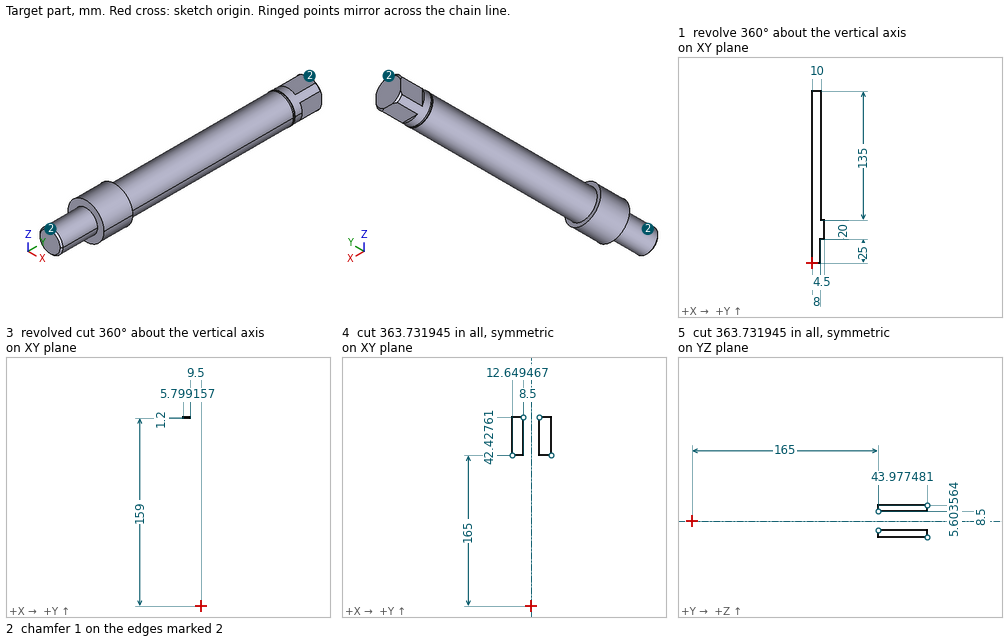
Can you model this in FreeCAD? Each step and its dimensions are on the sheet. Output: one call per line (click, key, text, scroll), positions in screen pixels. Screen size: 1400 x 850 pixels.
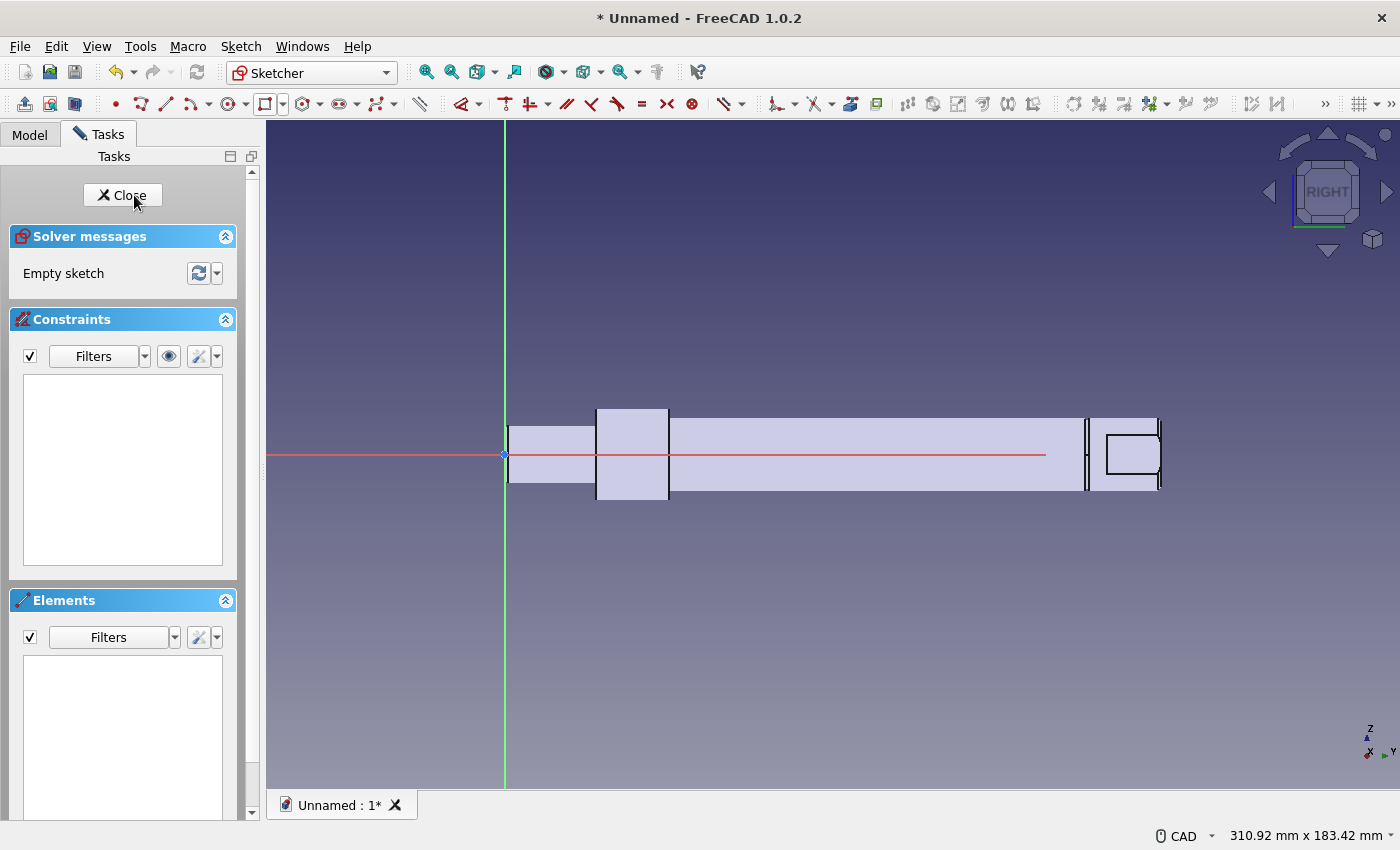
scroll(764, 454, down, 5)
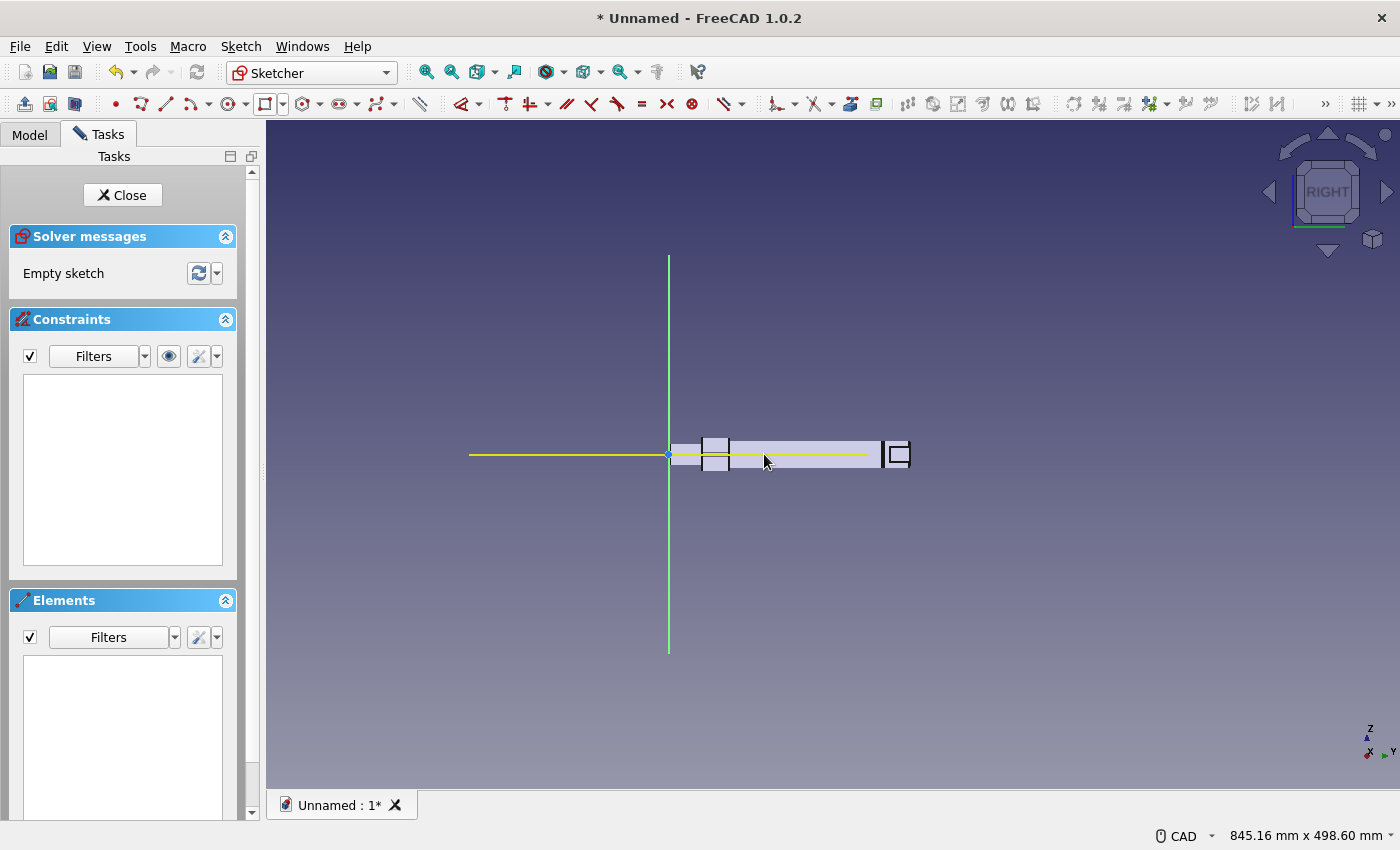
scroll(935, 454, up, 12)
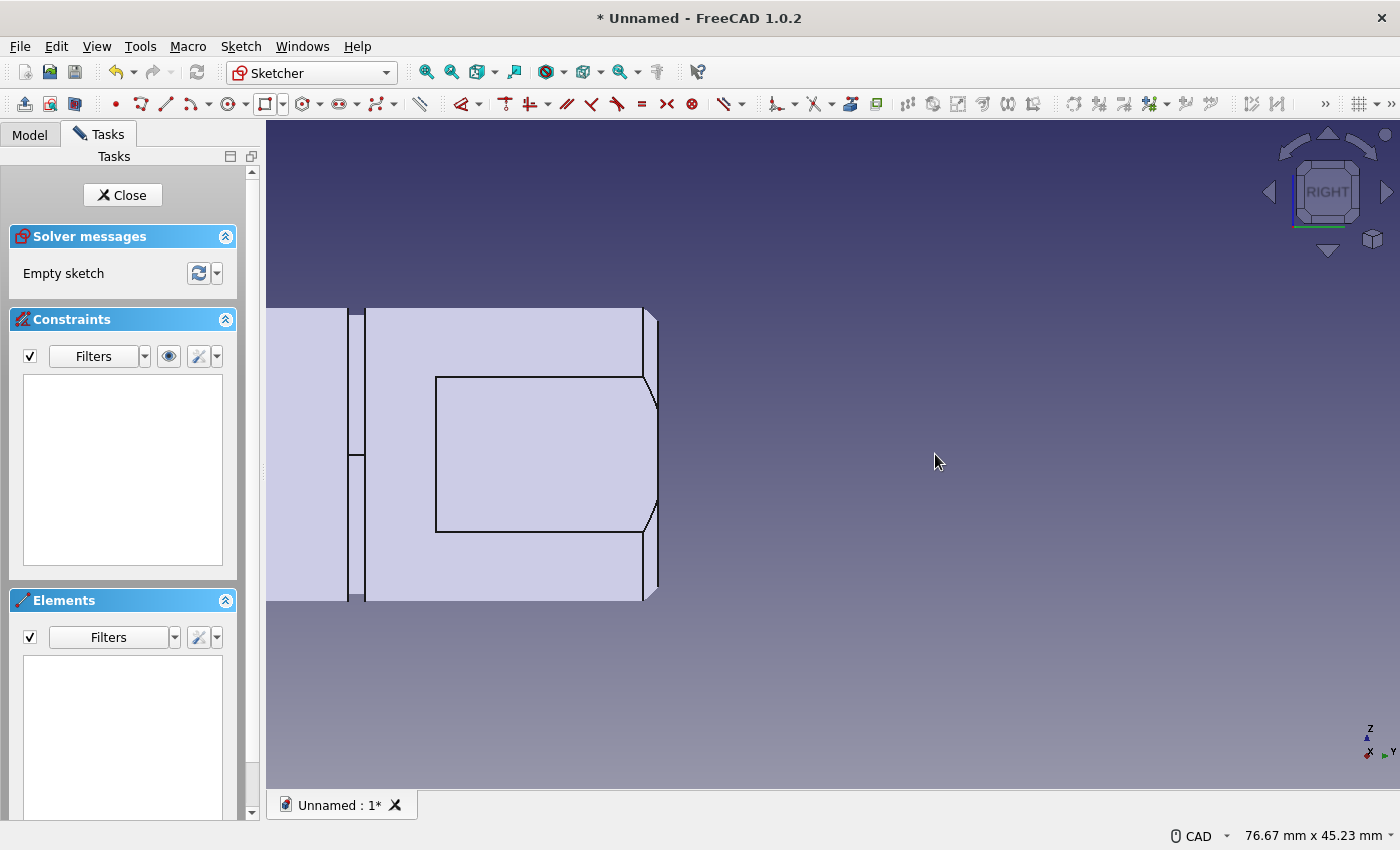
click(264, 104)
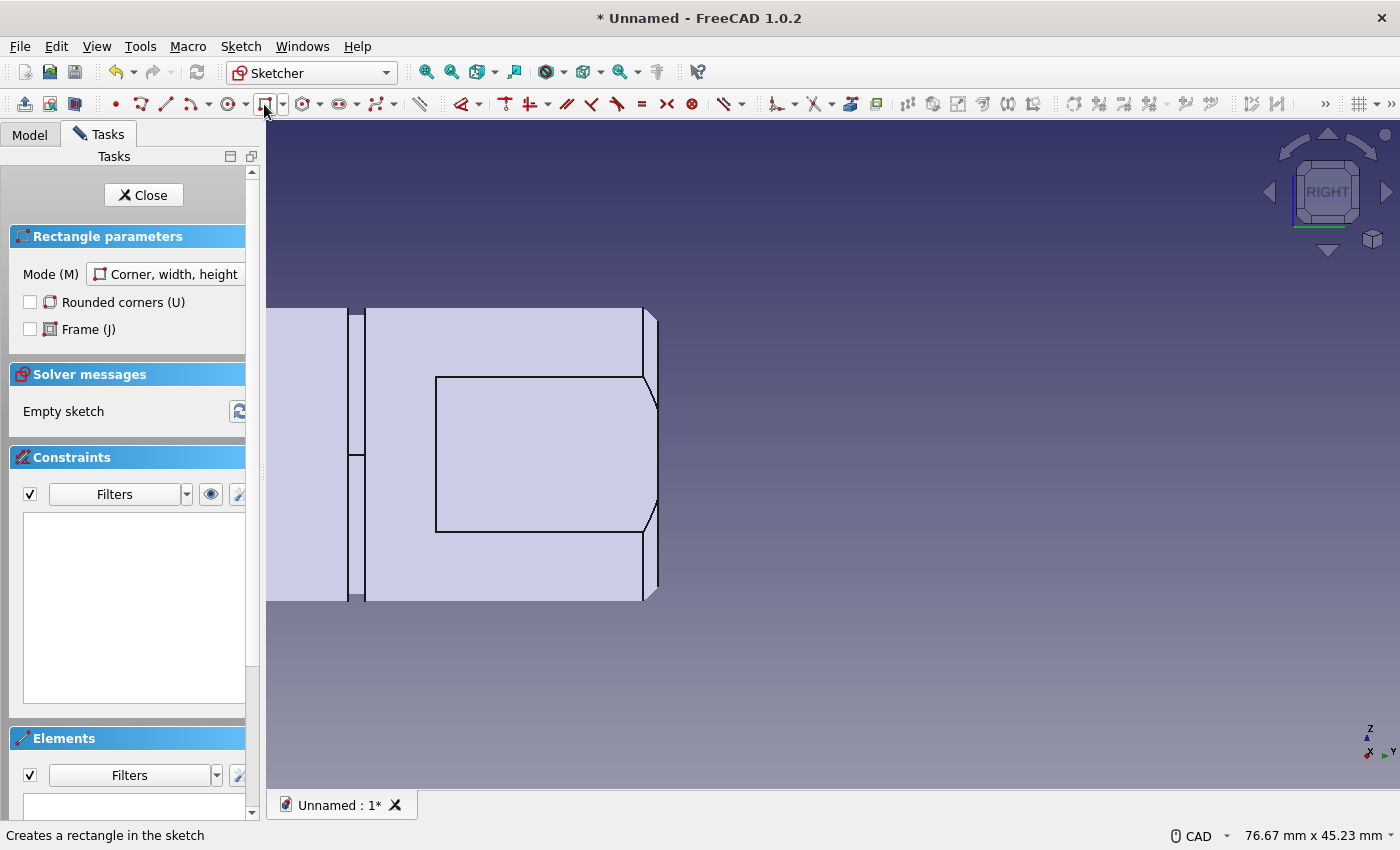
click(436, 246)
click(1087, 329)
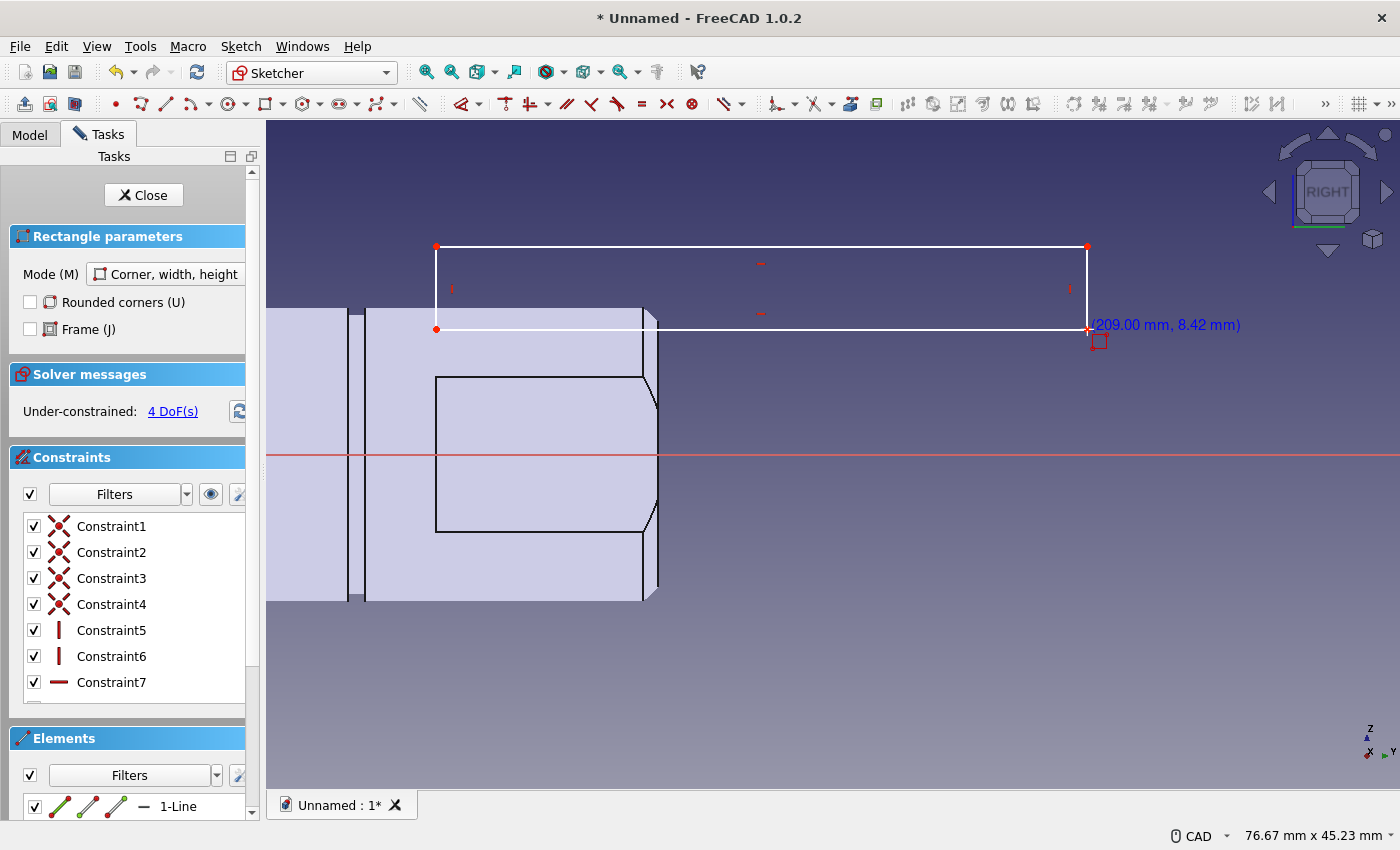
click(436, 580)
click(1087, 663)
key(Escape)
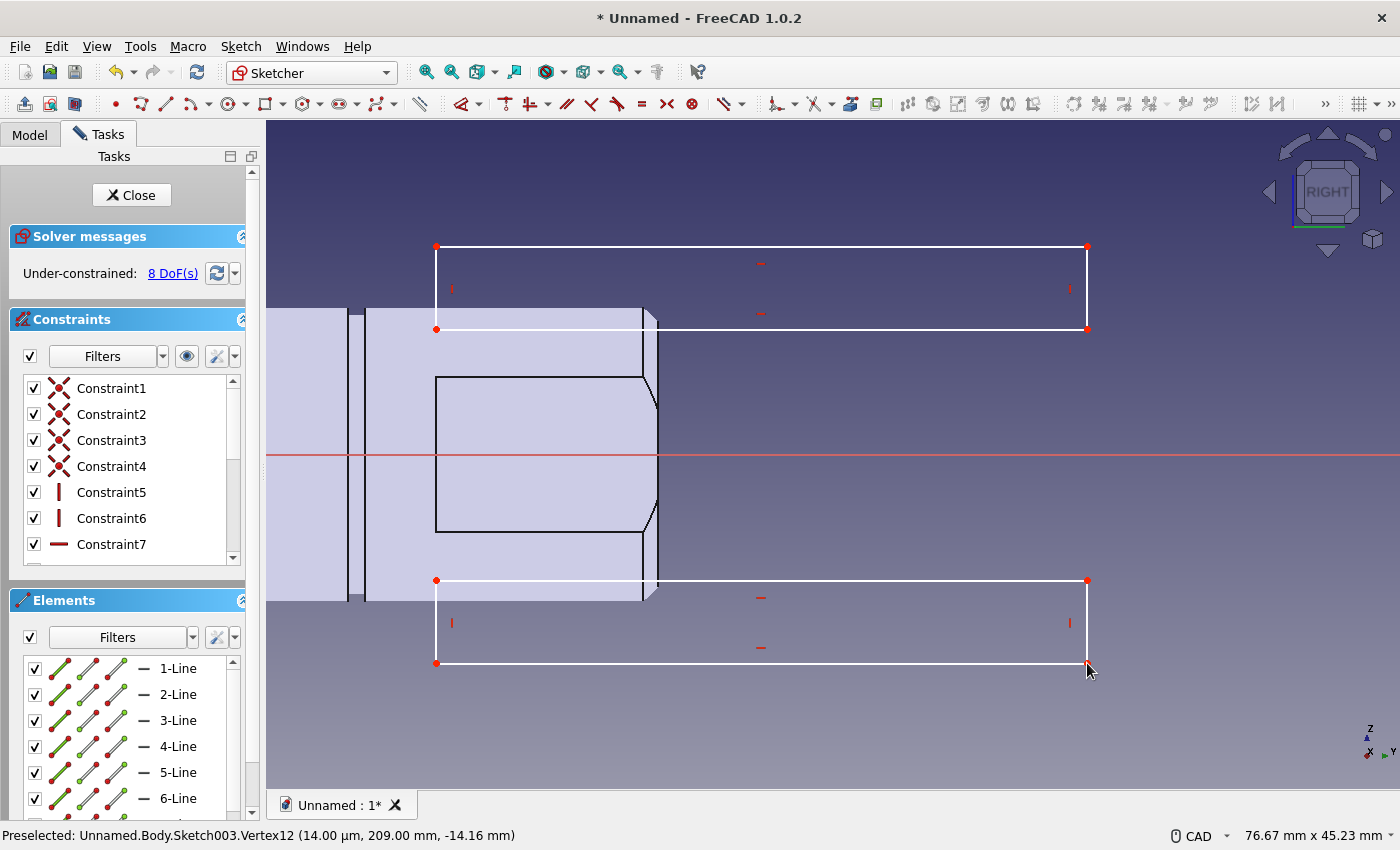
click(436, 330)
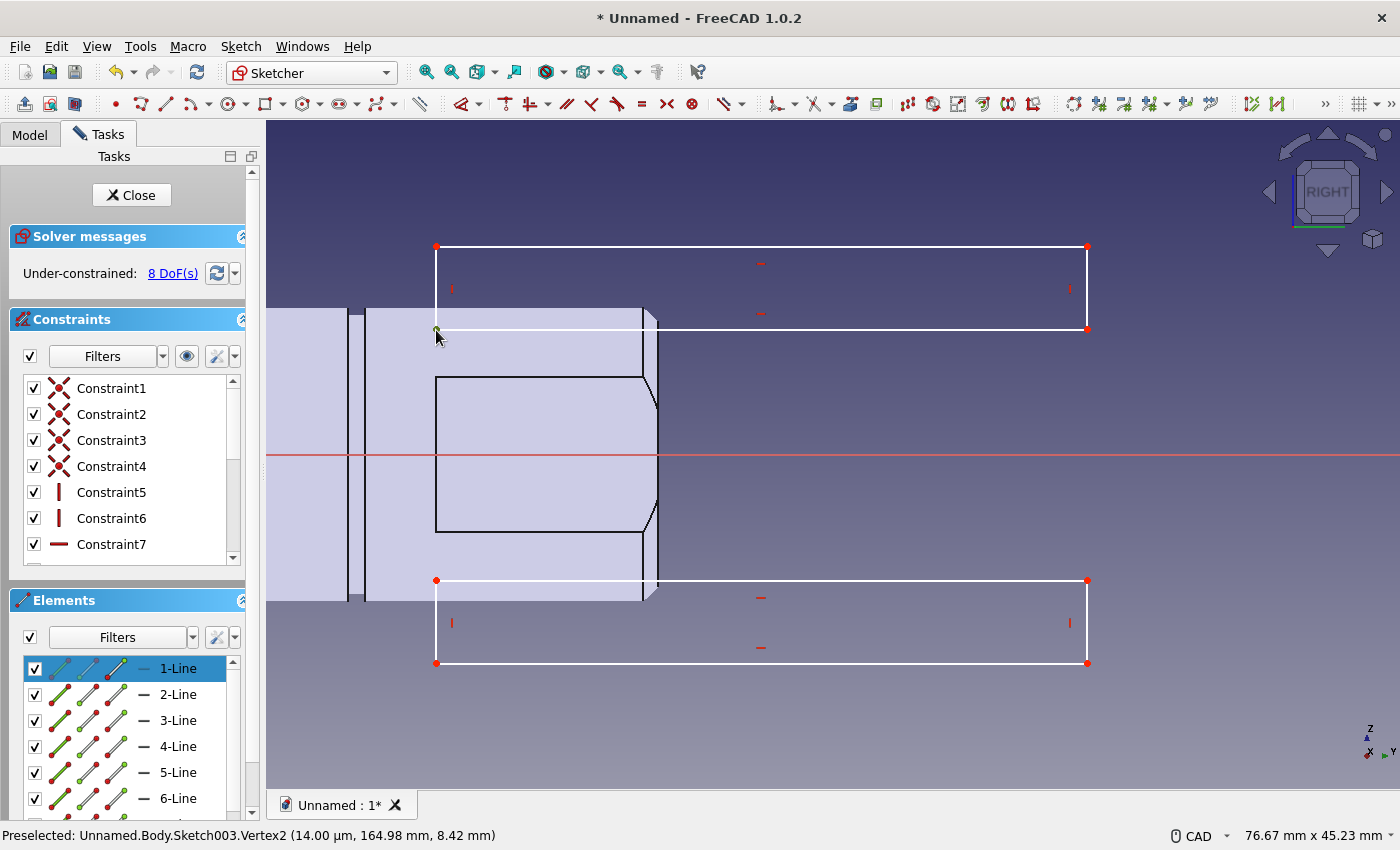
click(436, 581)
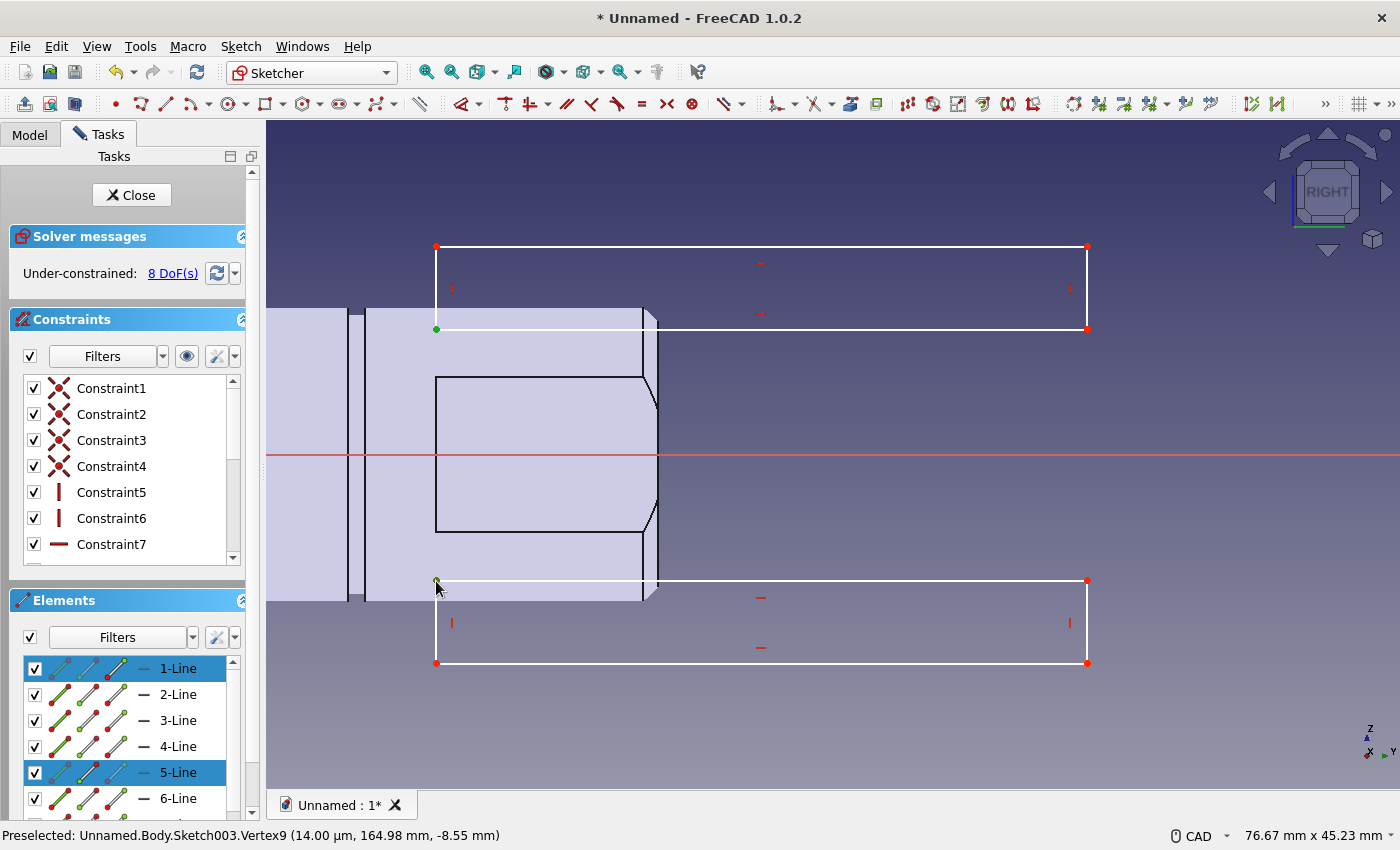
click(361, 454)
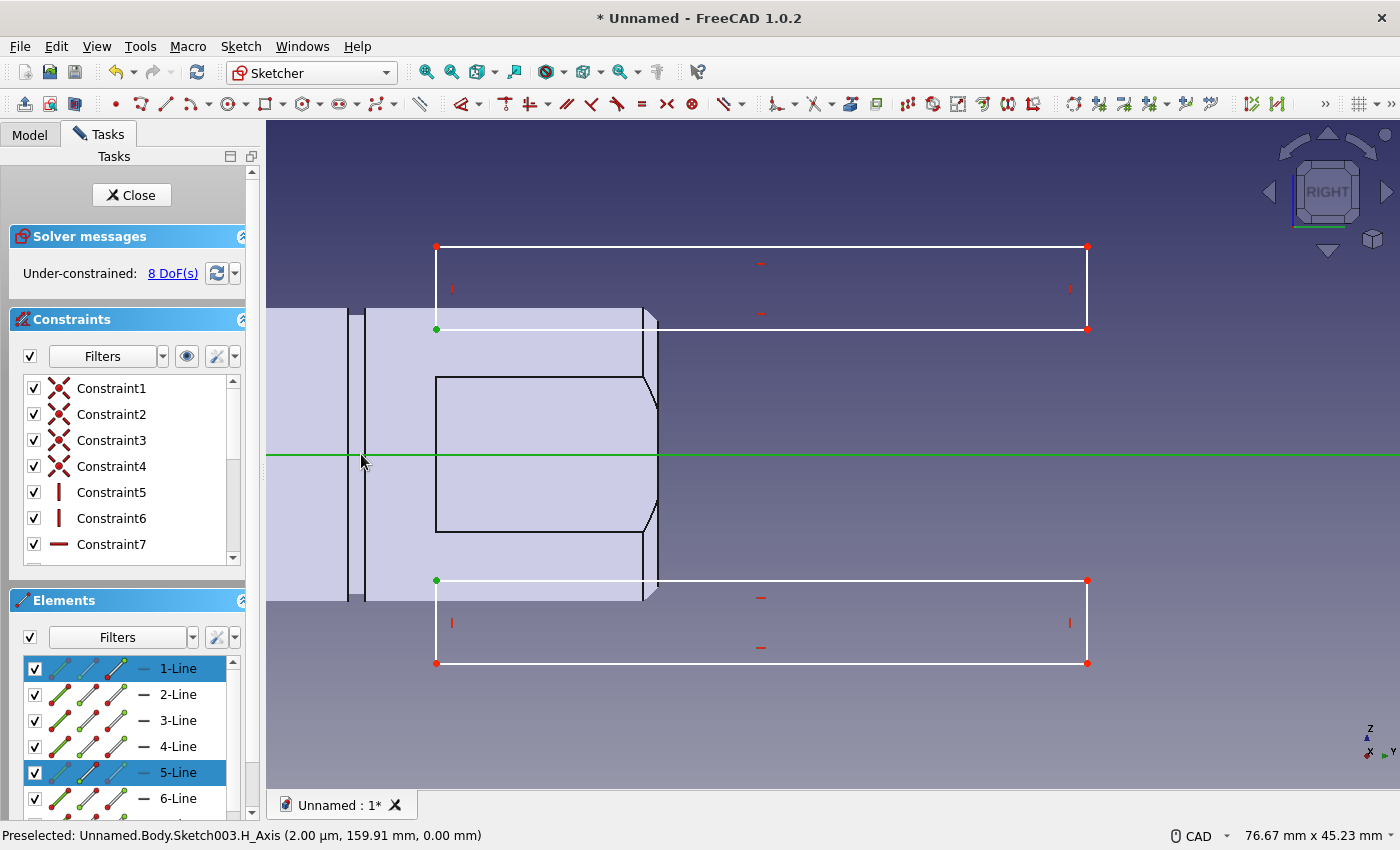
key(s)